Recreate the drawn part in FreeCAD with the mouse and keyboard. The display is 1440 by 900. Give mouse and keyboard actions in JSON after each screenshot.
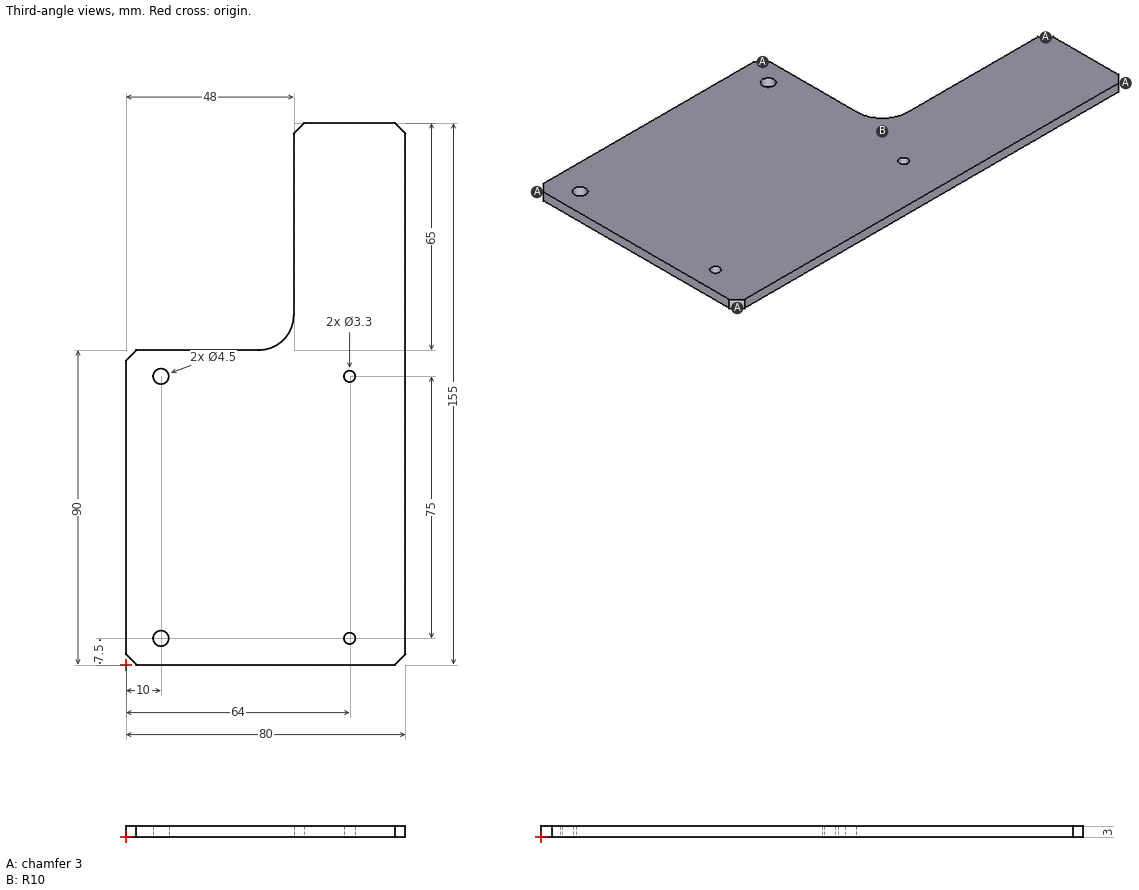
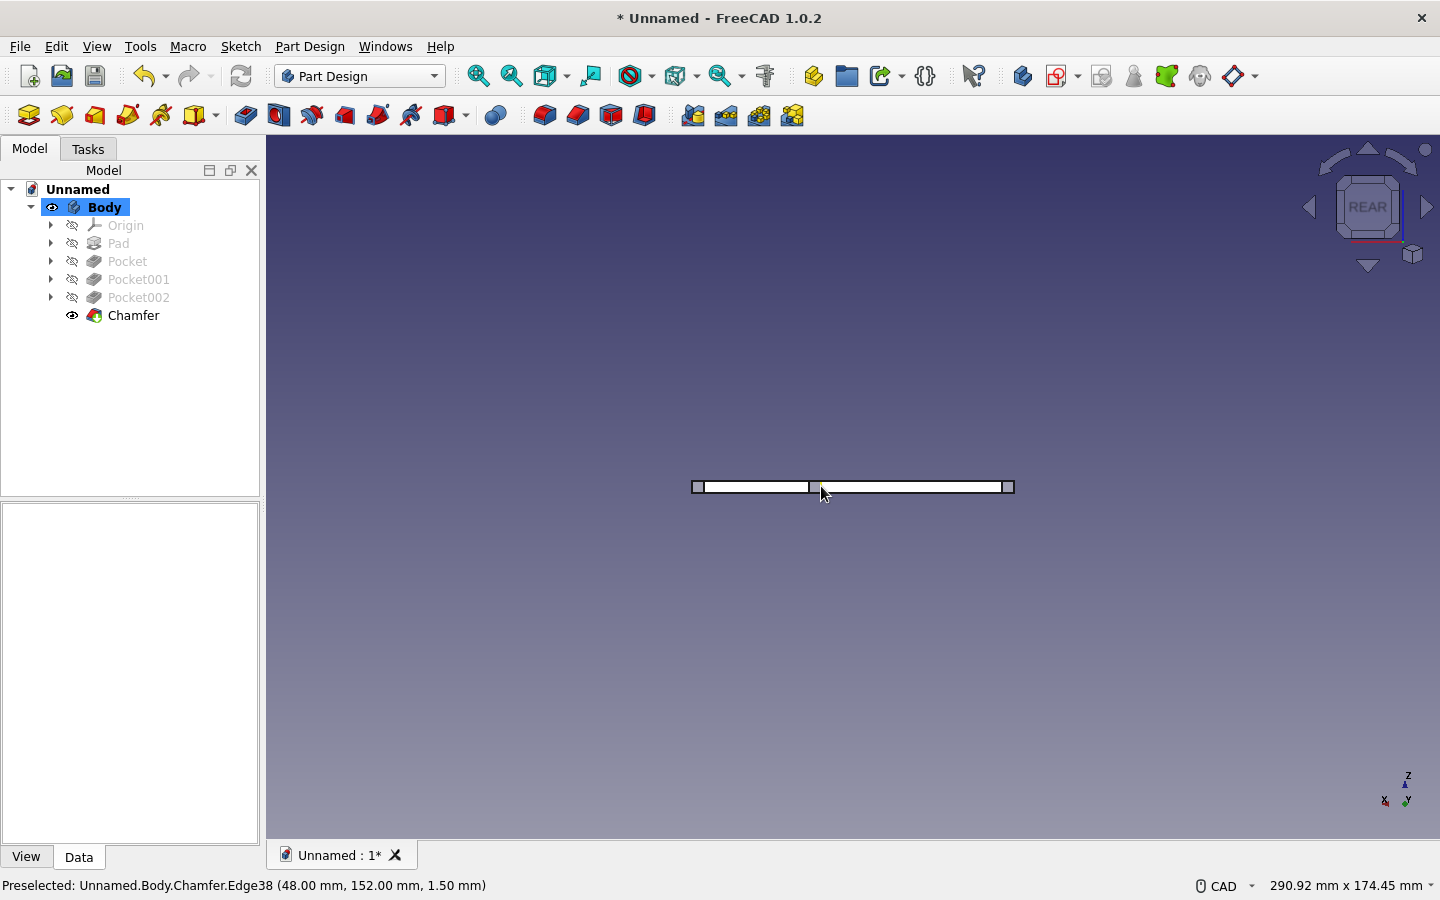
{"action": "key", "text": "6"}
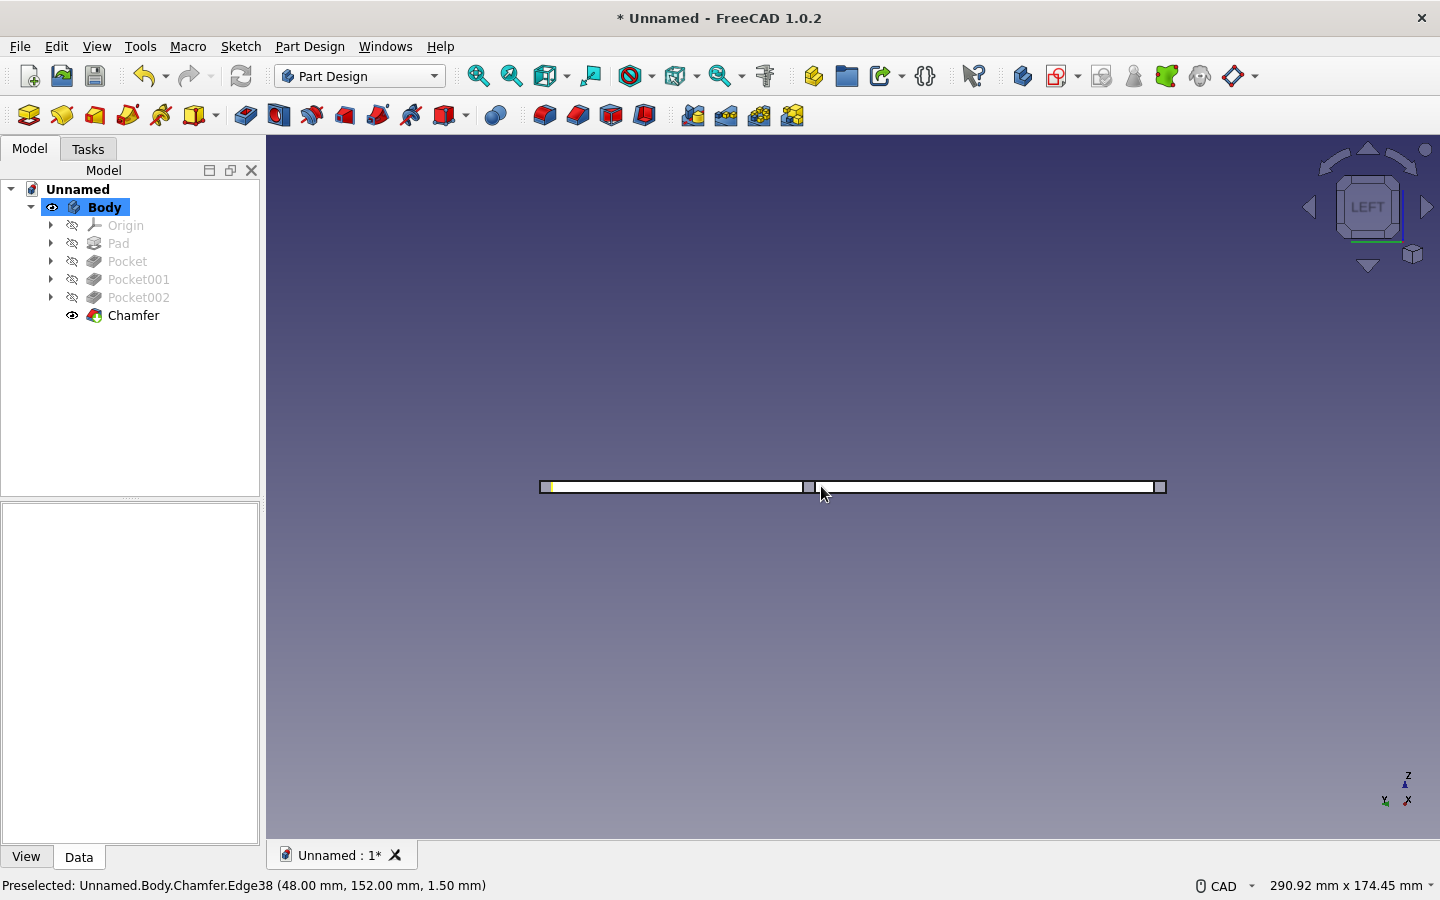
{"action": "scroll", "coordinate": [803, 486], "scroll_direction": "up", "scroll_amount": 6}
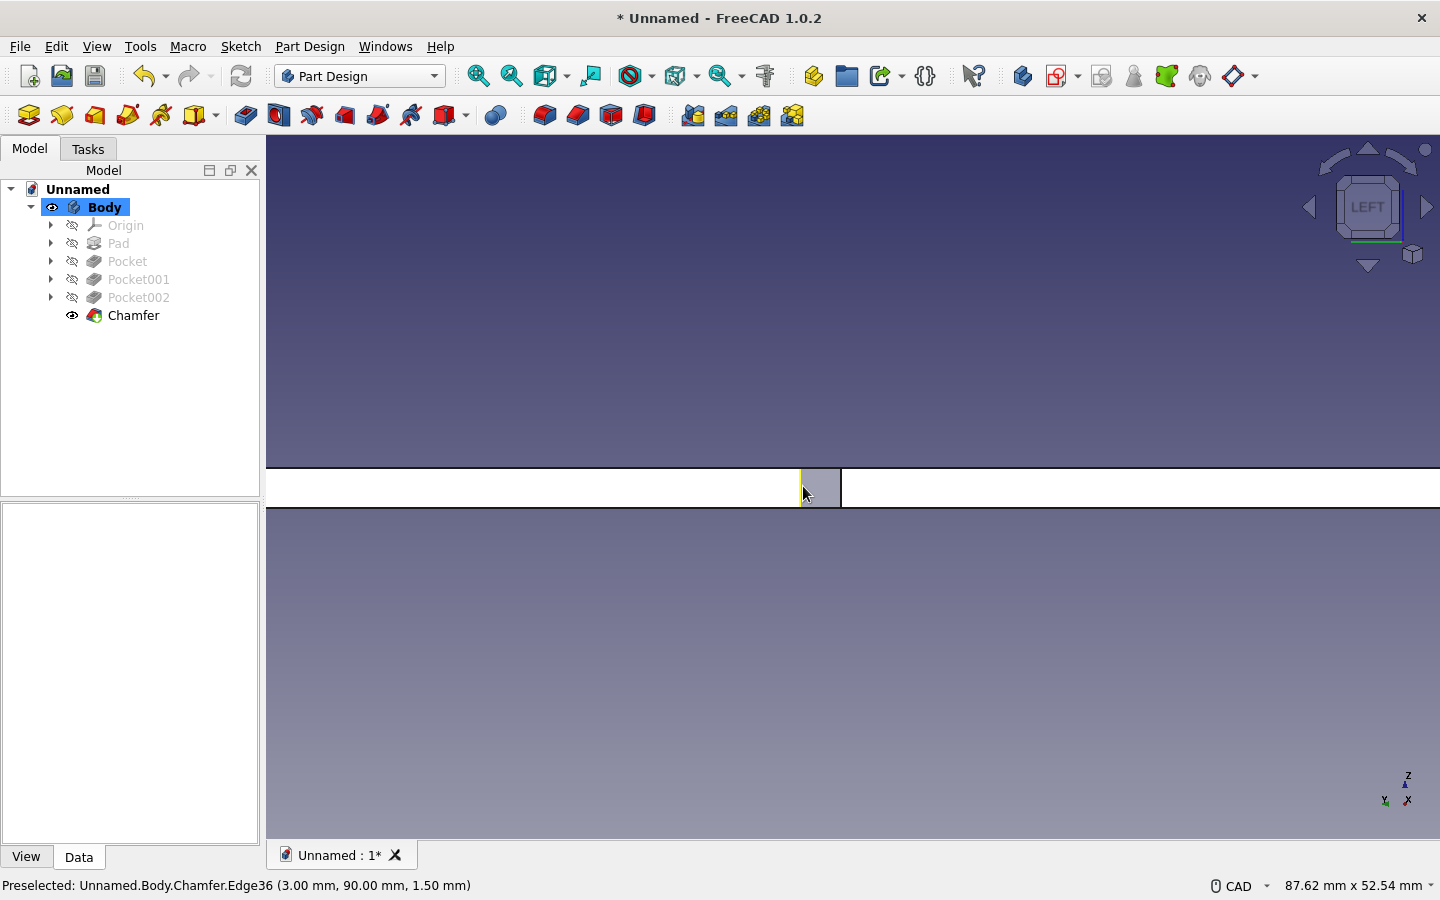
{"action": "left_click", "coordinate": [479, 76]}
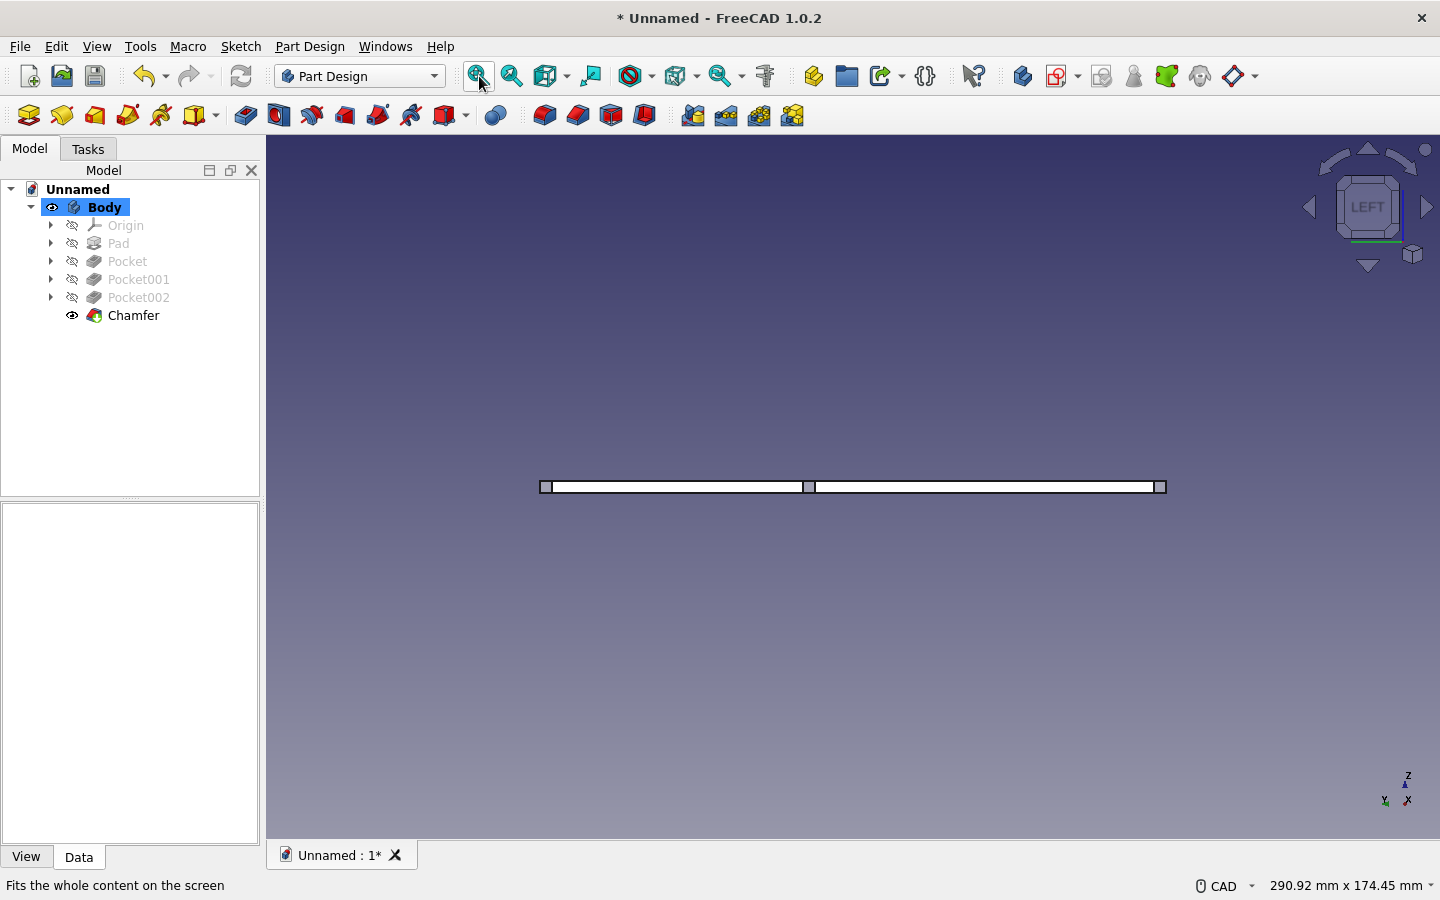
{"action": "key", "text": "v 3"}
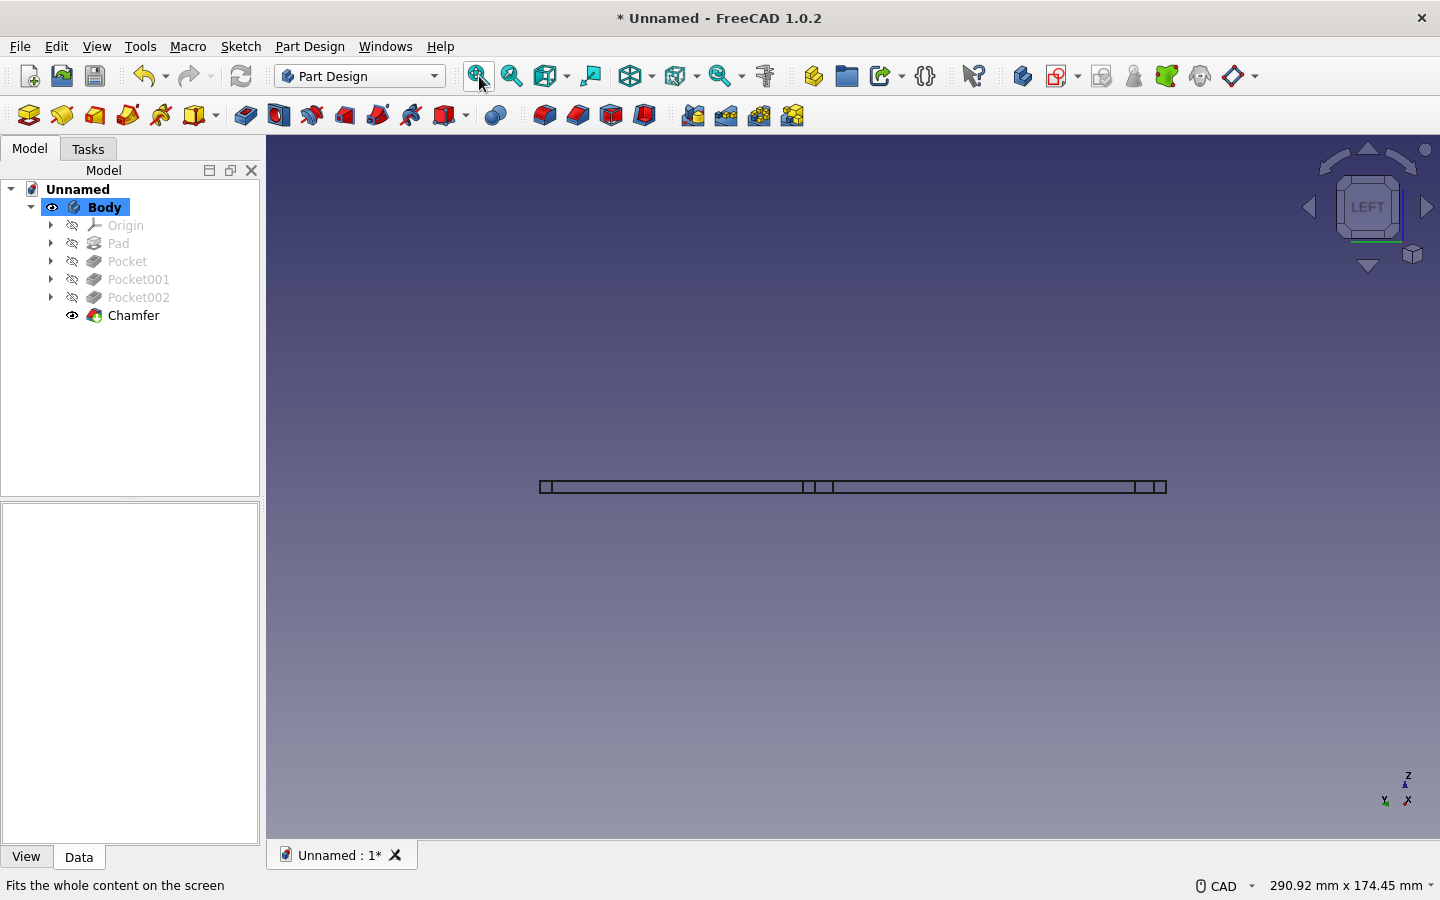
{"action": "key", "text": "0"}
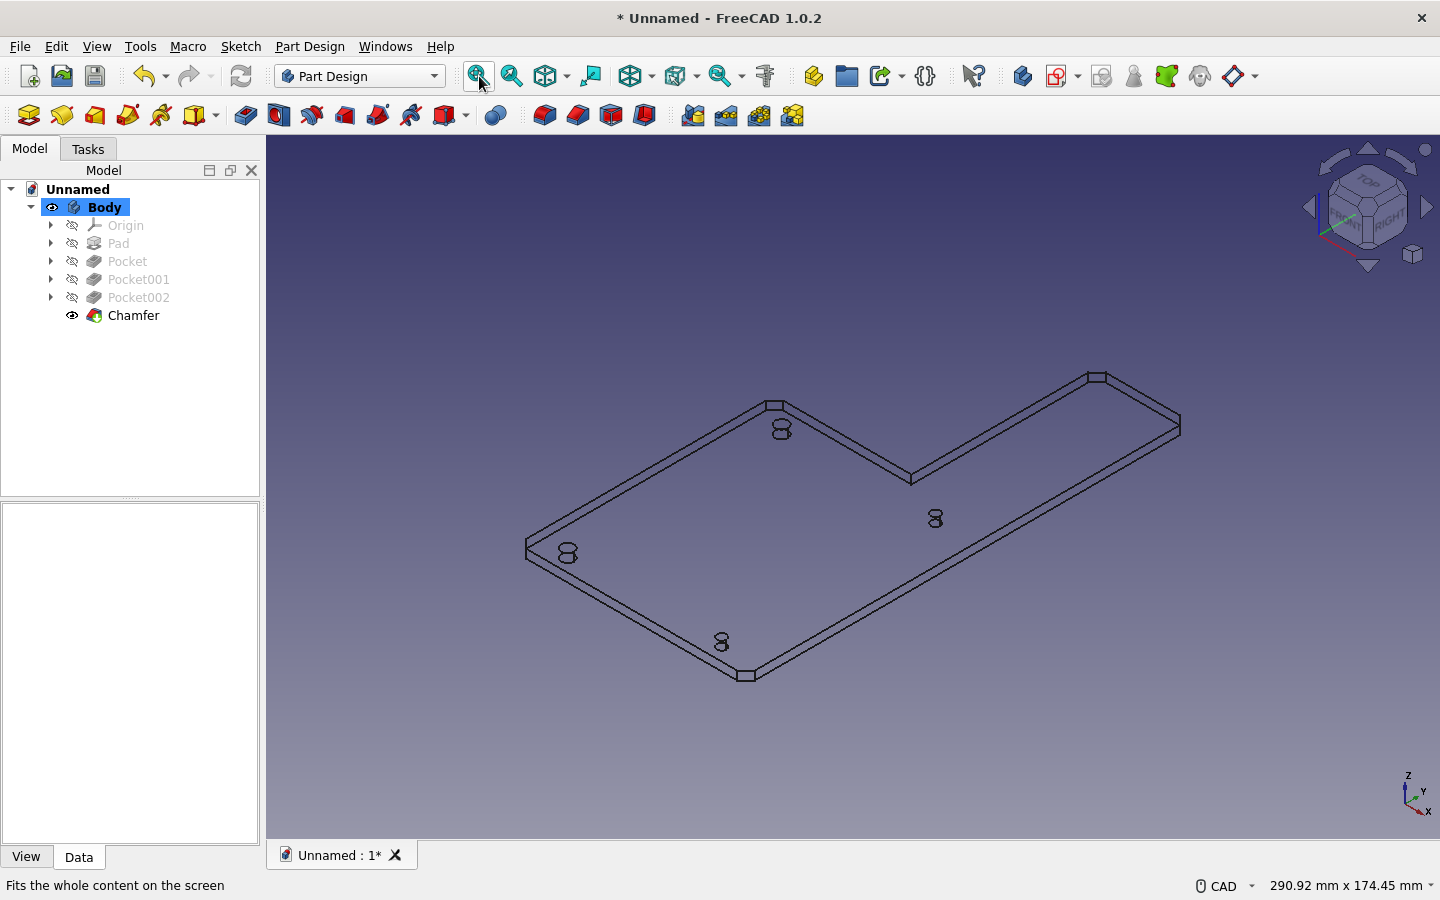
{"action": "left_click", "coordinate": [911, 480]}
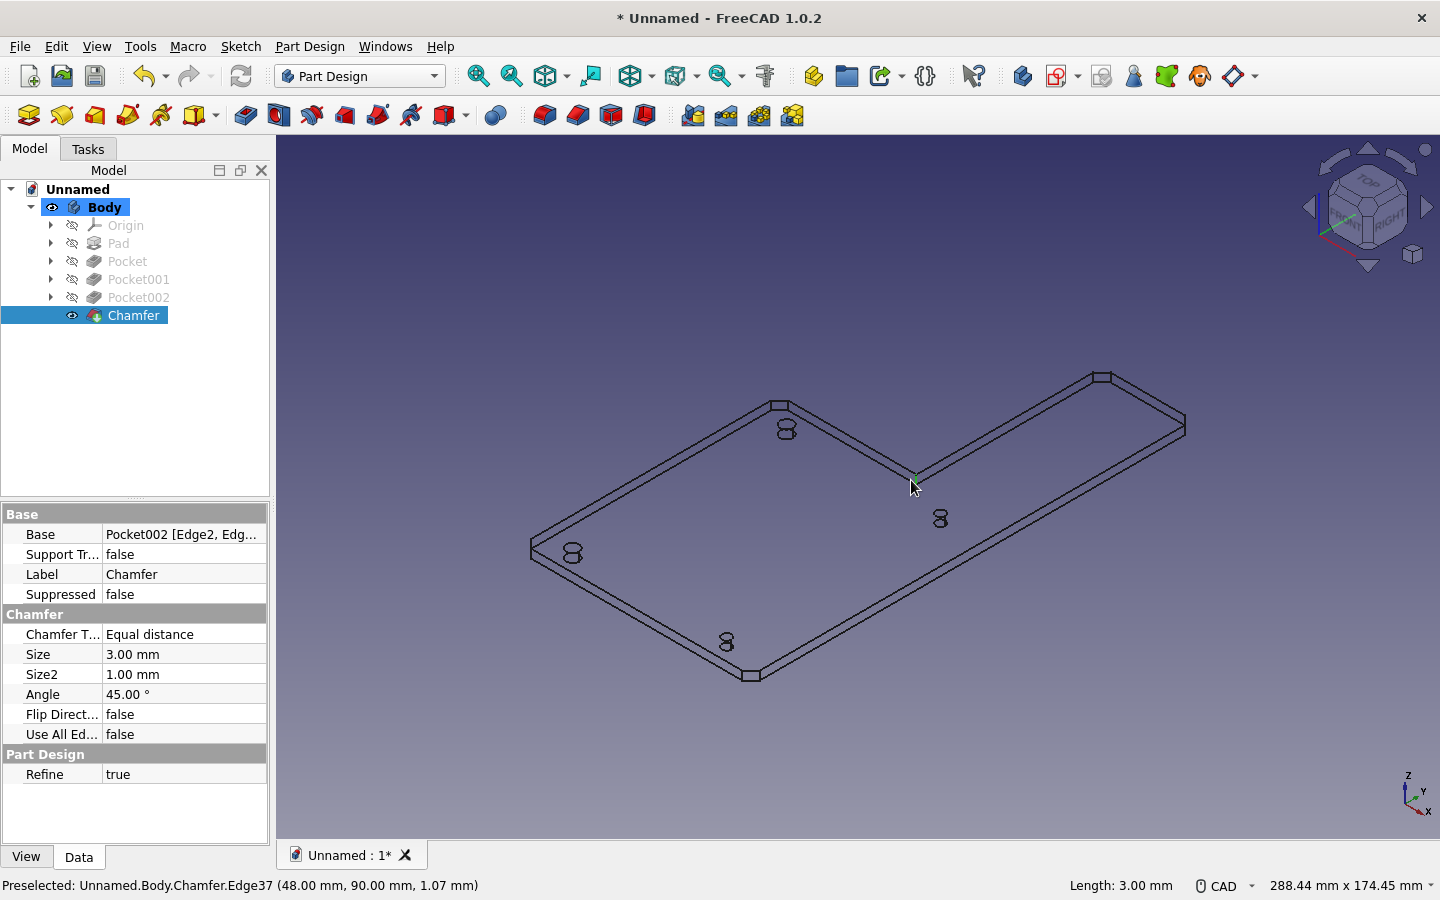
{"action": "key", "text": "v 1"}